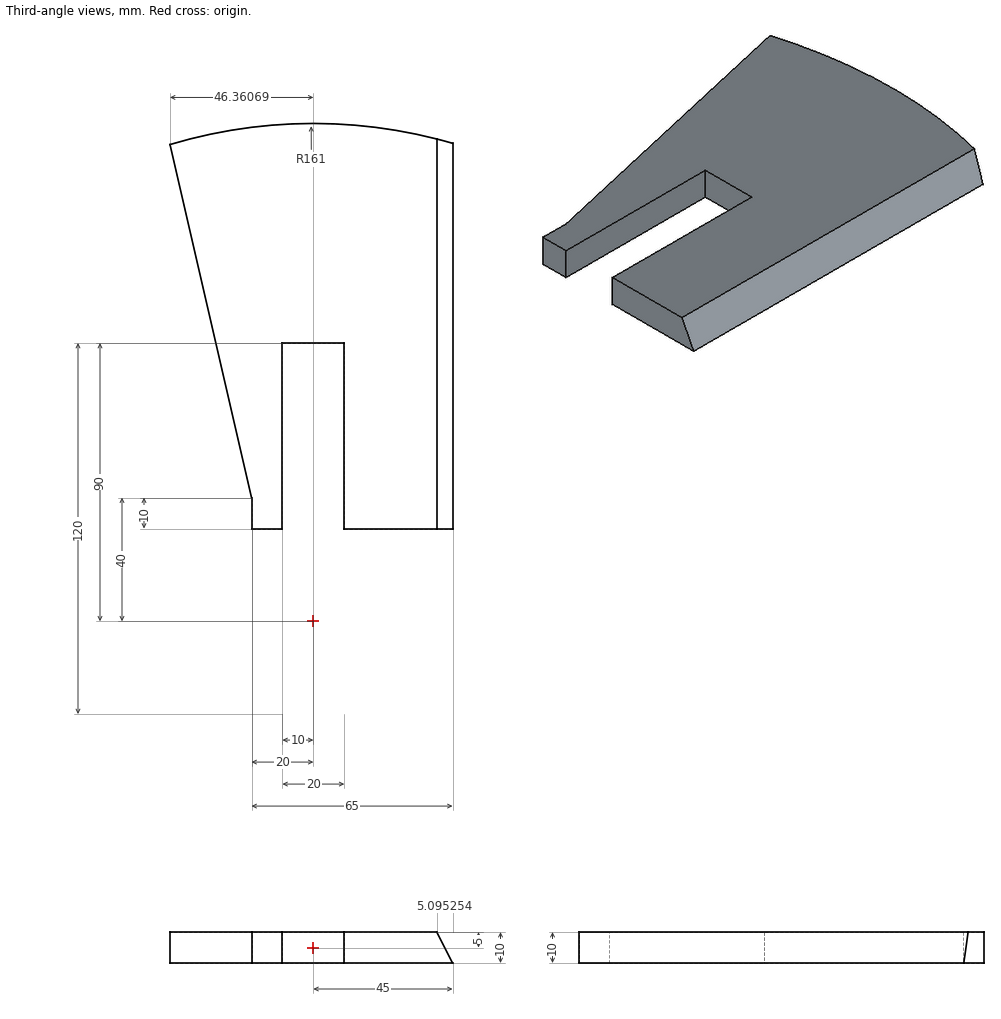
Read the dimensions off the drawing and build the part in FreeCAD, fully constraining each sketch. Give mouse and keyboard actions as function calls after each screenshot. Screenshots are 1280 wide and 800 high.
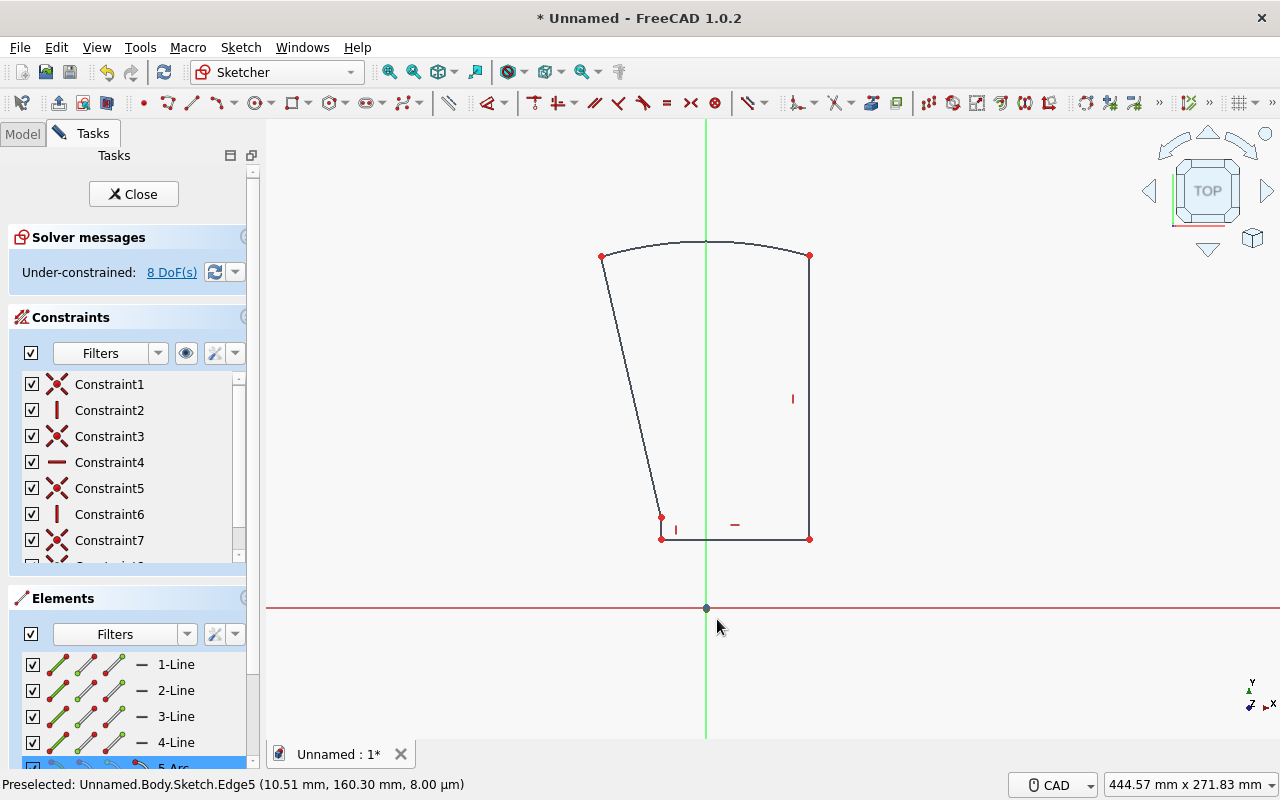
click(534, 104)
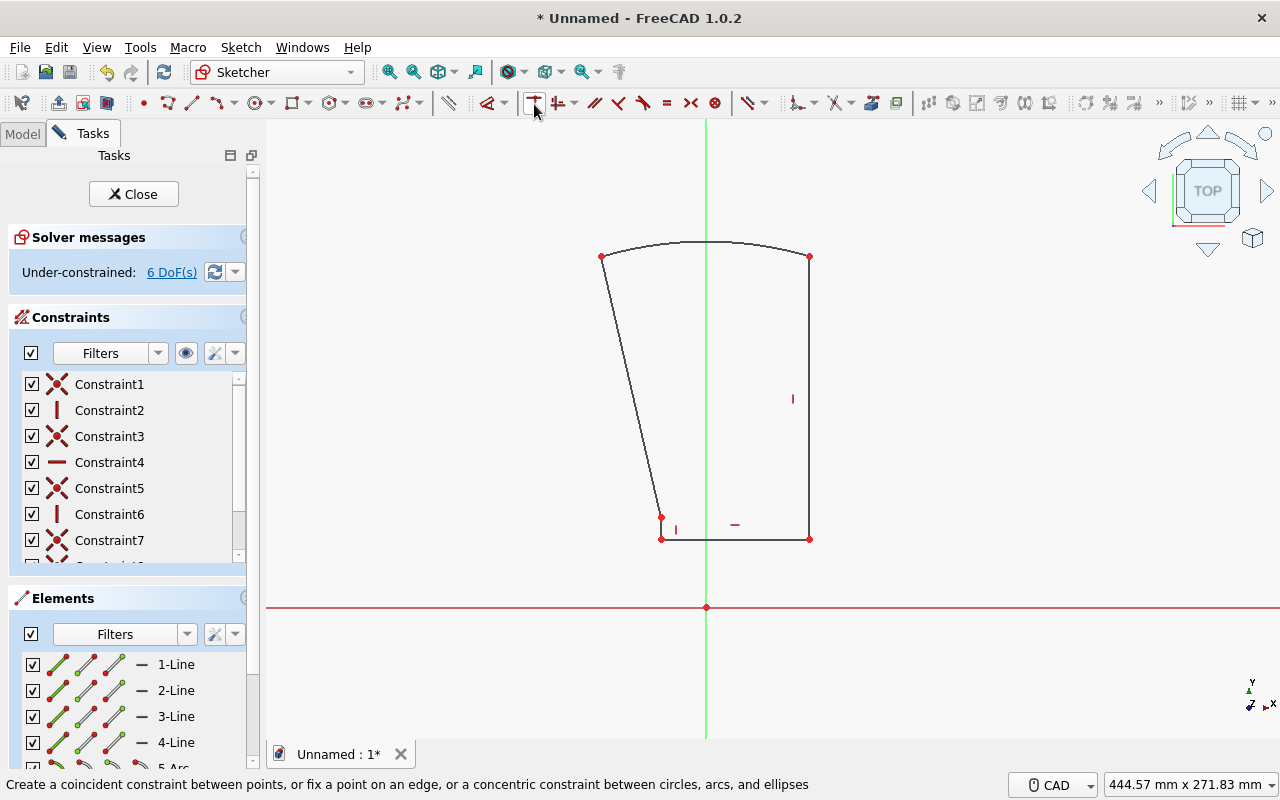
click(488, 104)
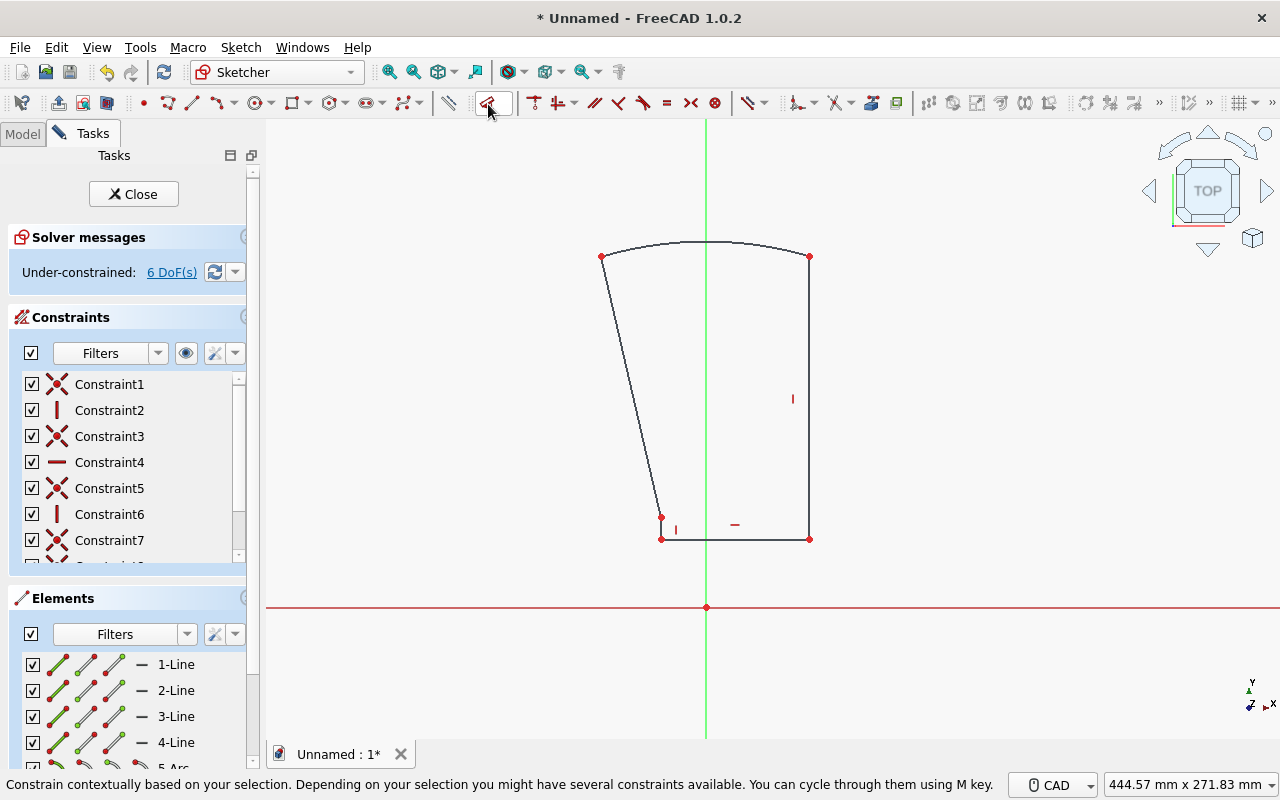
click(747, 244)
click(751, 212)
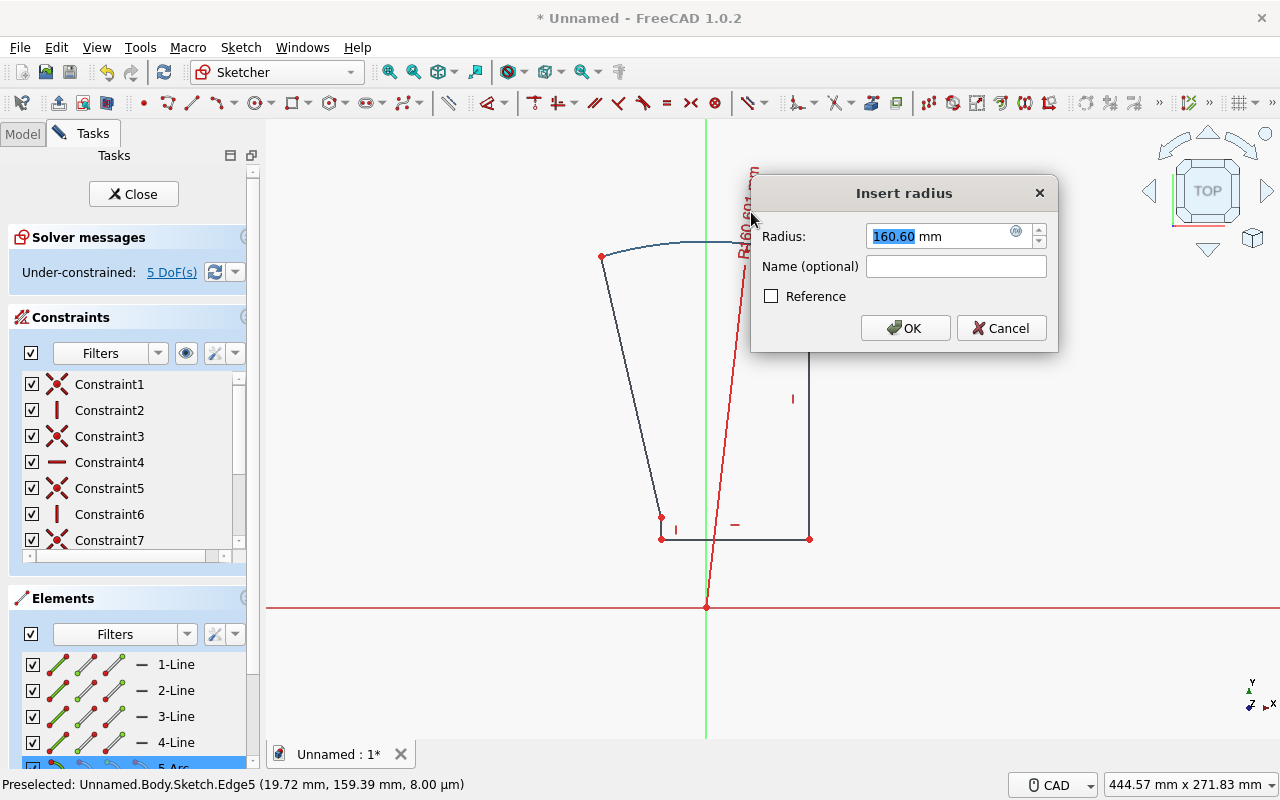
text(161)
key(Return)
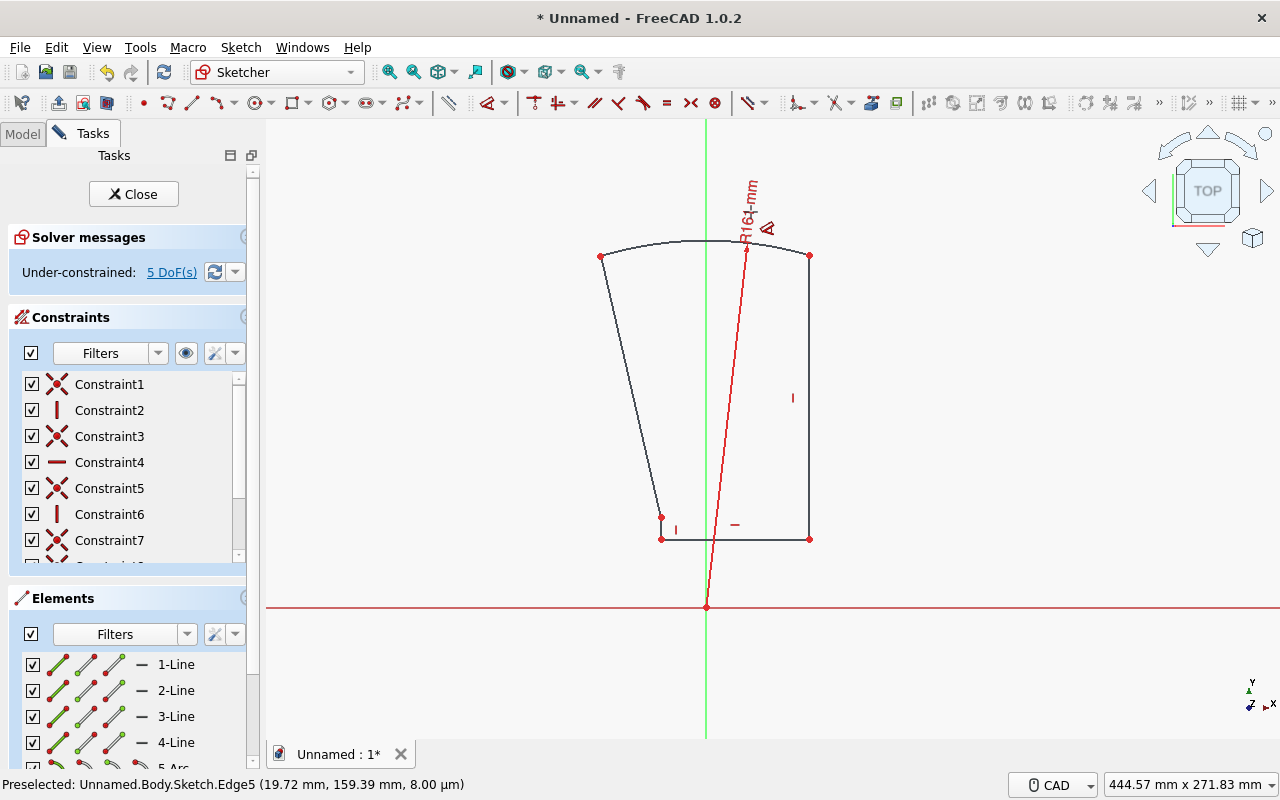
scroll(661, 529, up, 3)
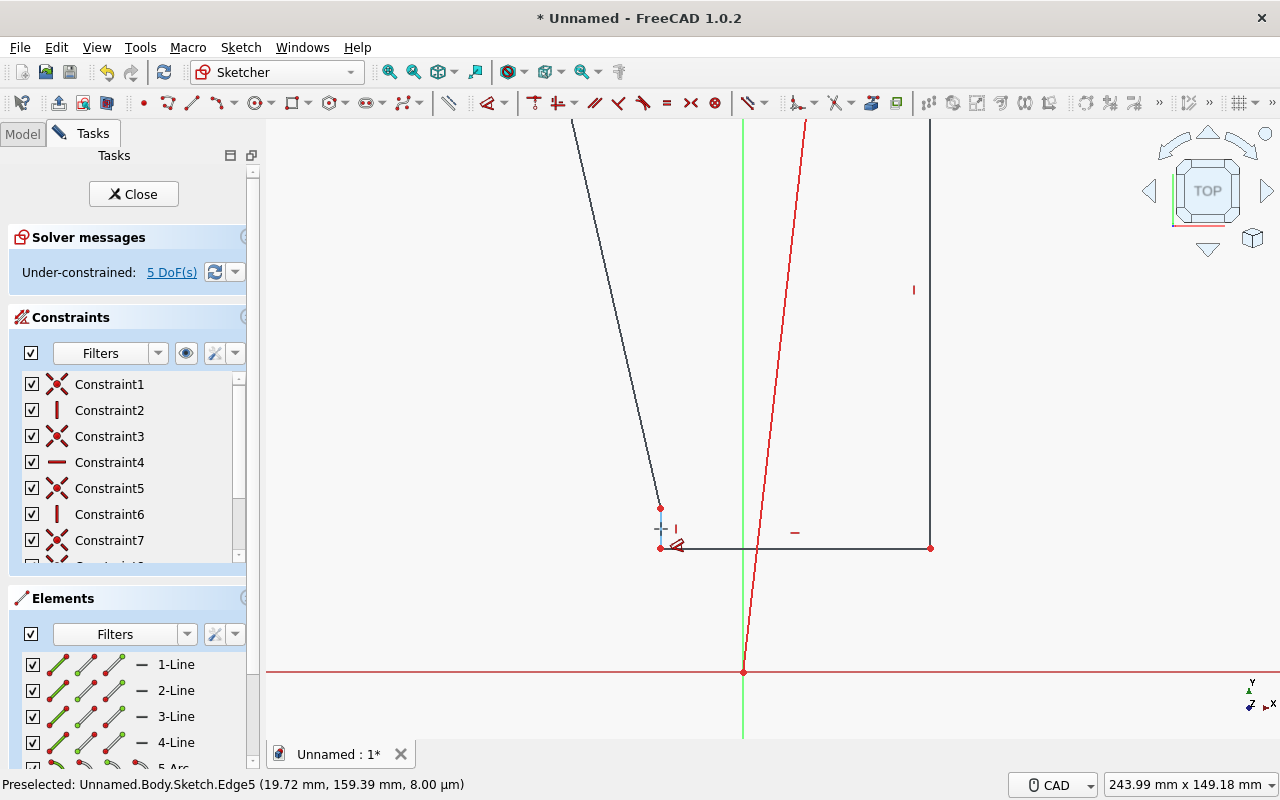
click(661, 528)
click(627, 528)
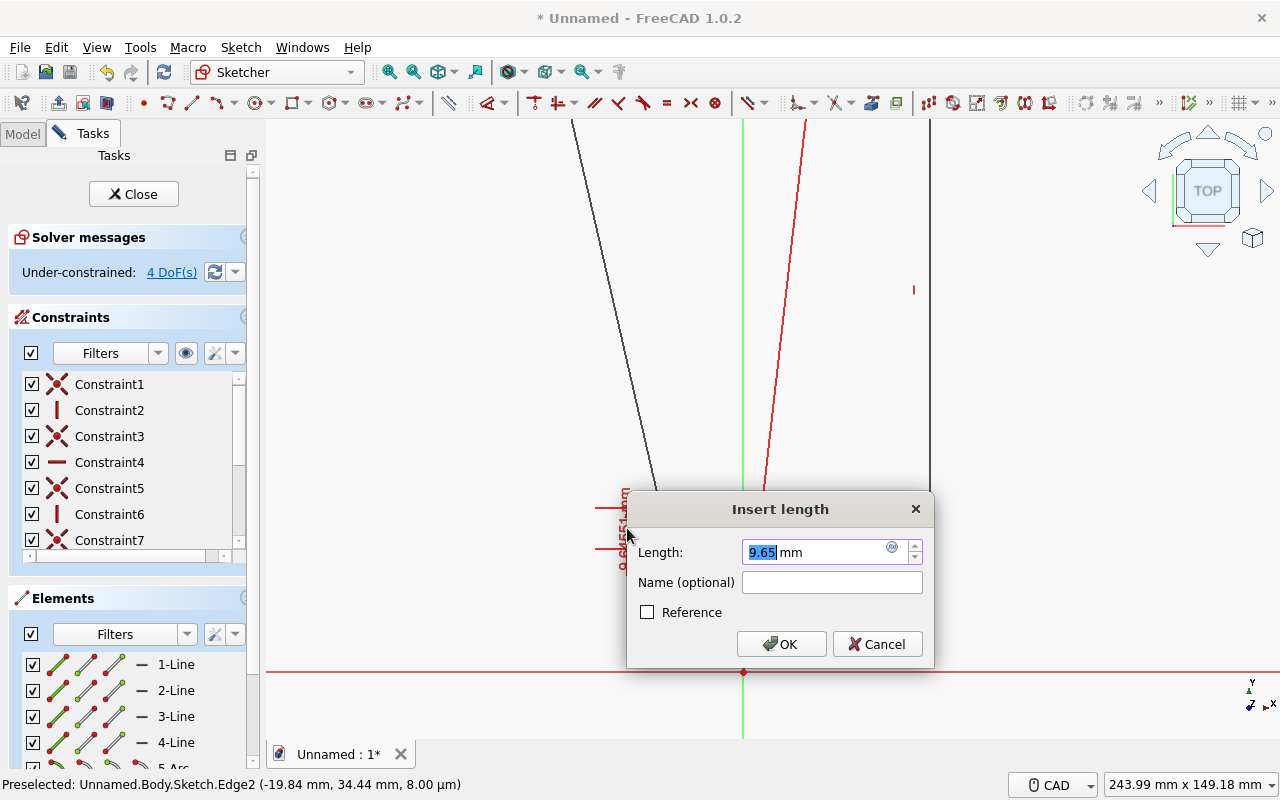
text(10)
key(Return)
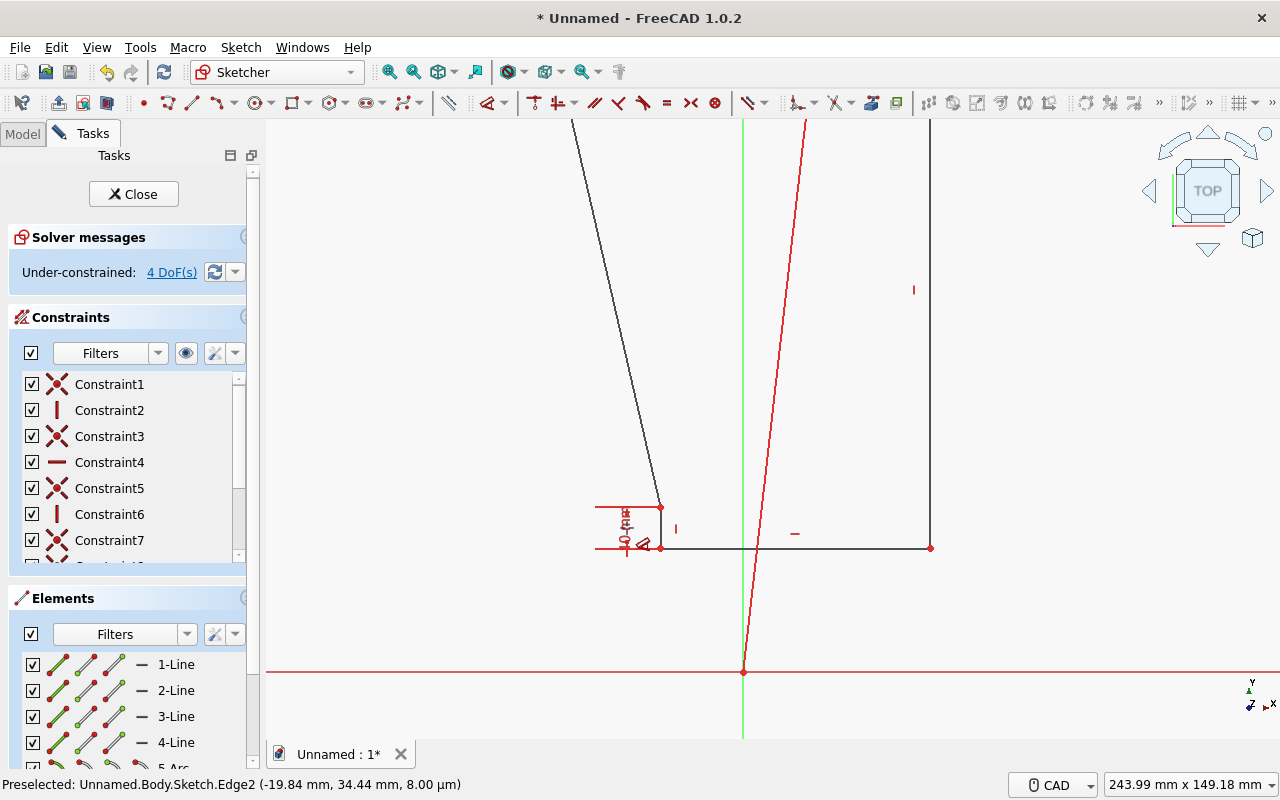
click(742, 549)
click(796, 583)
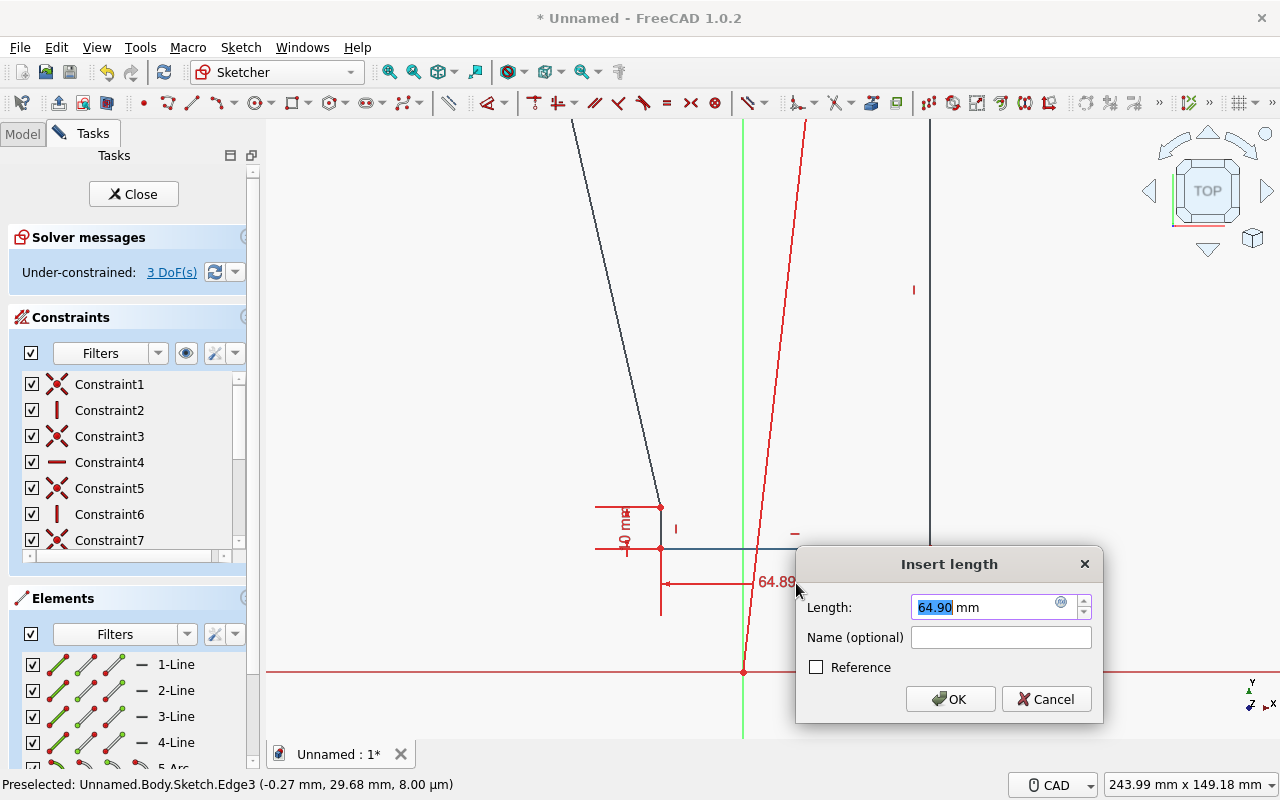
text(65)
key(Return)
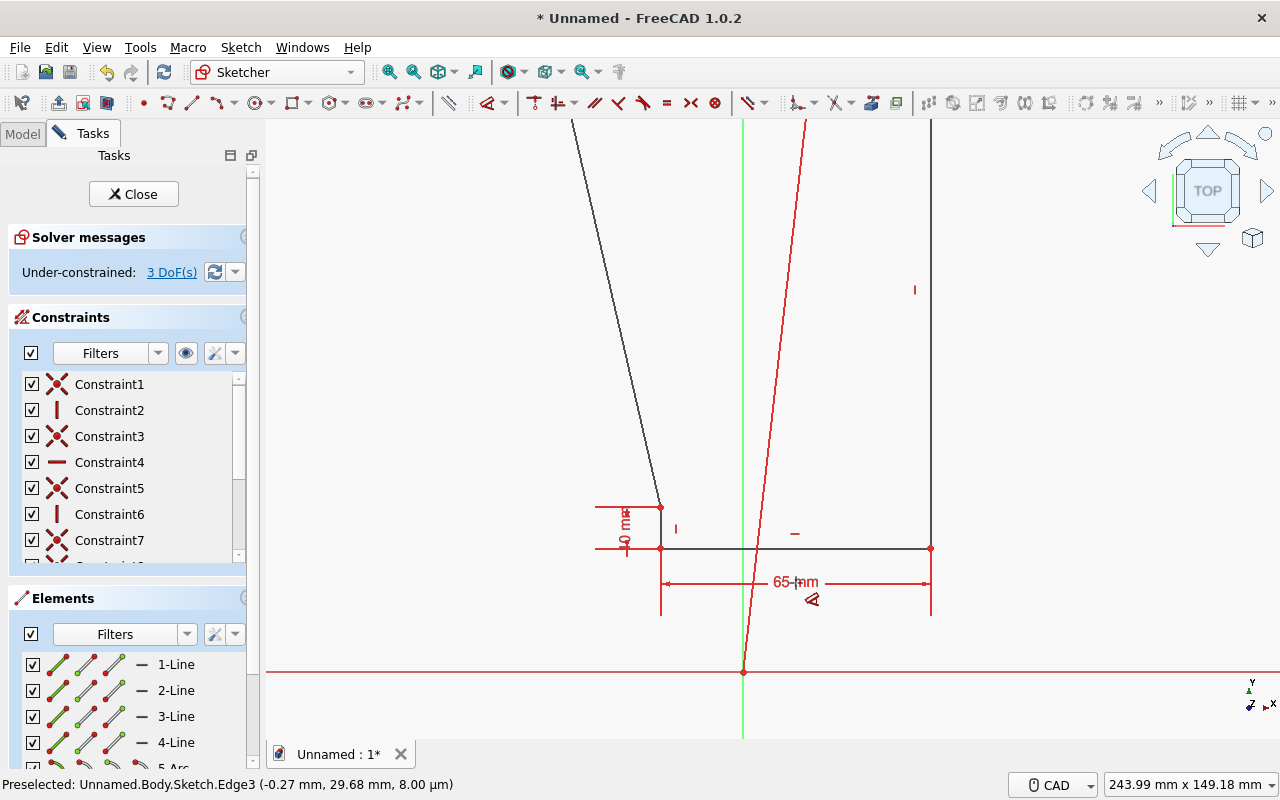
click(661, 507)
click(702, 706)